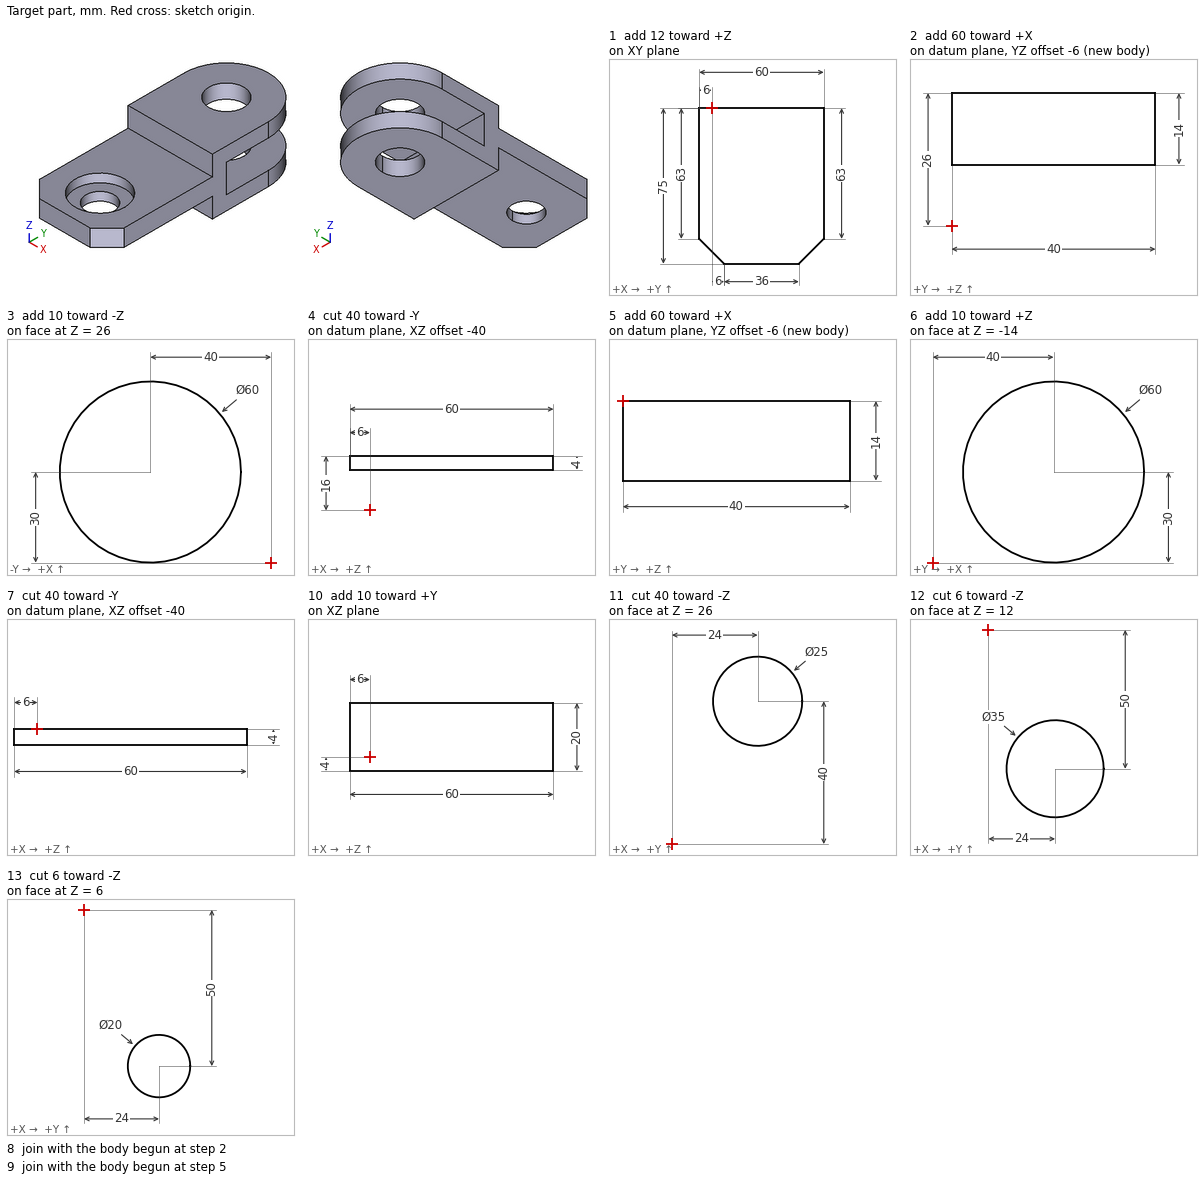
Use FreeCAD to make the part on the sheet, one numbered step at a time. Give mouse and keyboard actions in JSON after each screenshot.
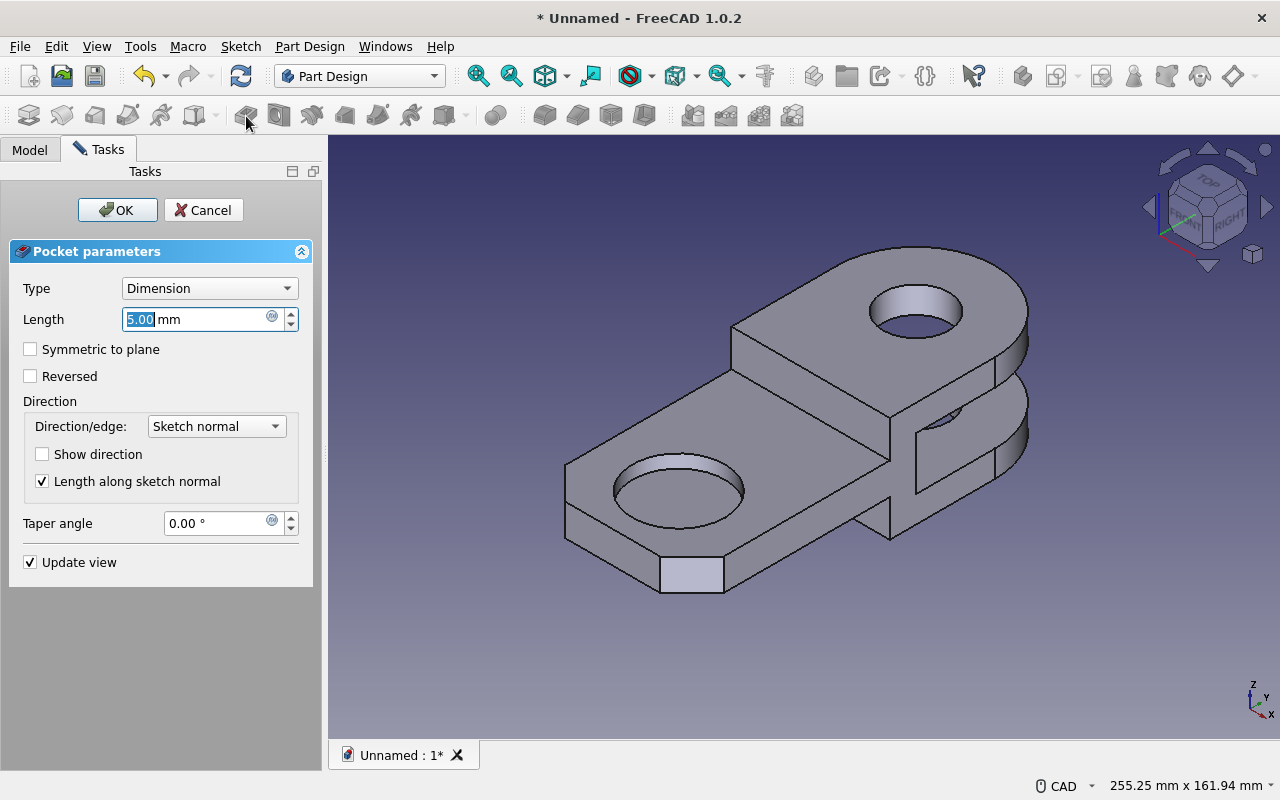
{"action": "type", "text": "6"}
{"action": "key", "text": "Tab"}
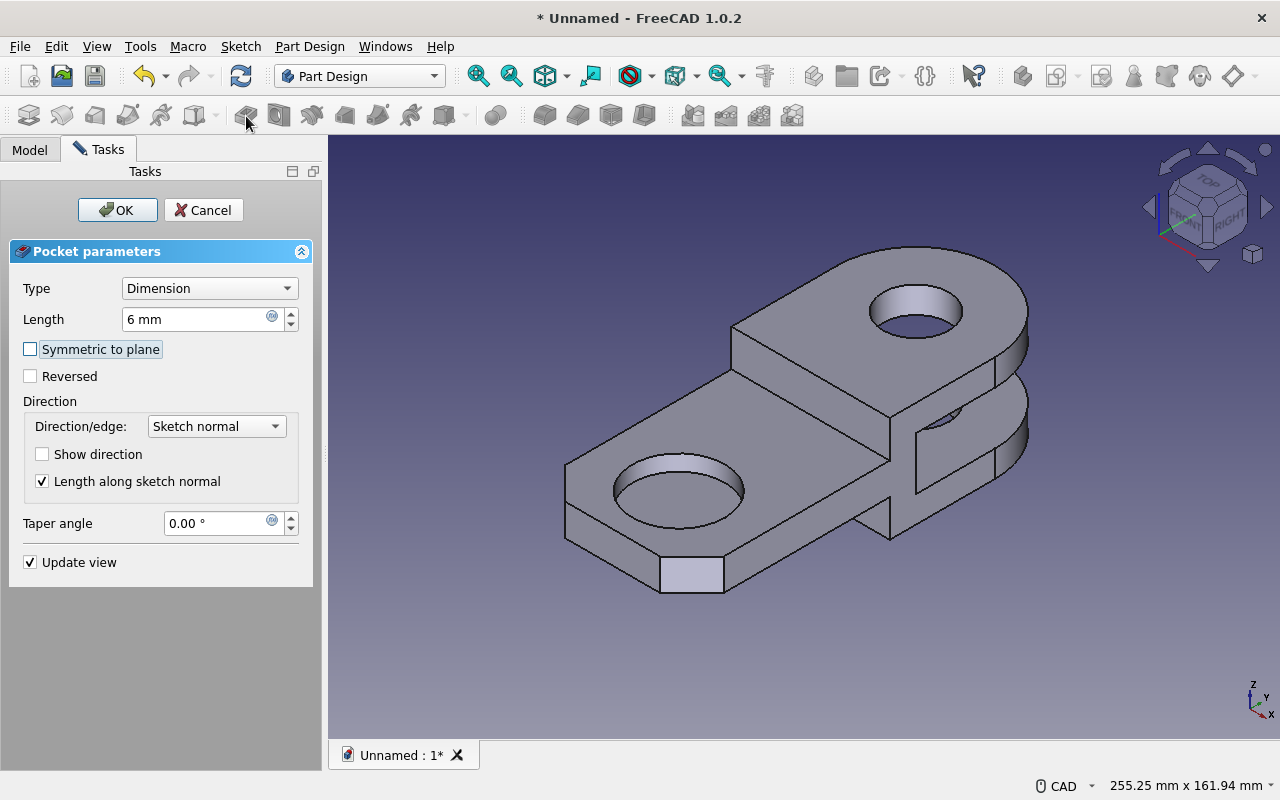
{"action": "left_click", "coordinate": [118, 210]}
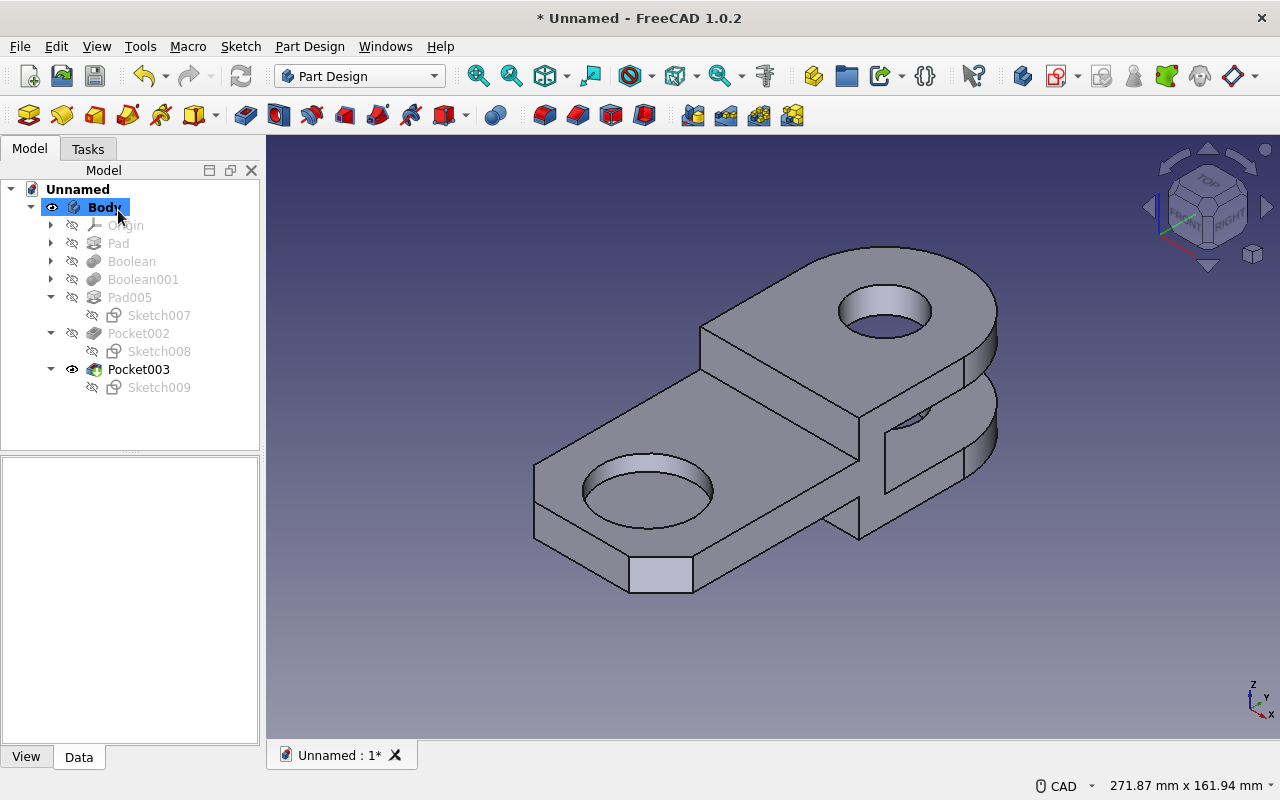
{"action": "left_click", "coordinate": [648, 508]}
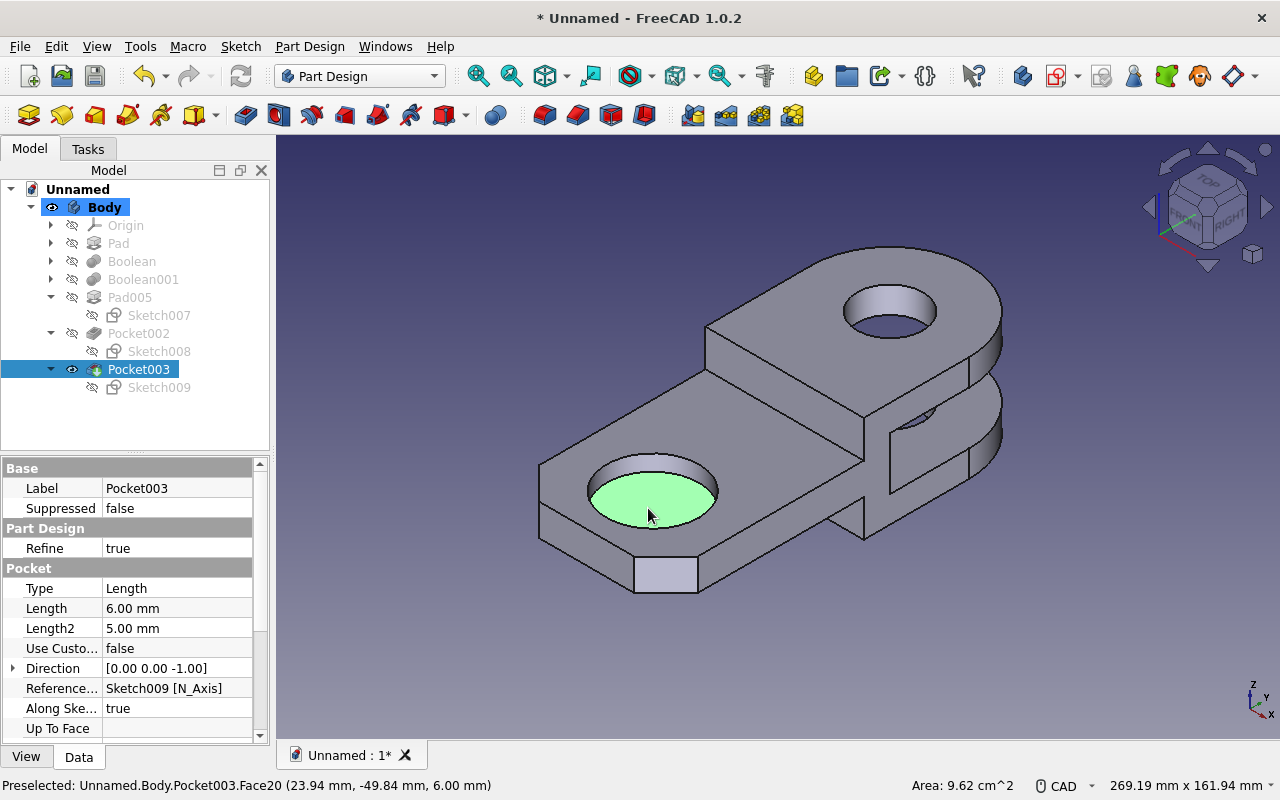
{"action": "left_click", "coordinate": [1056, 76]}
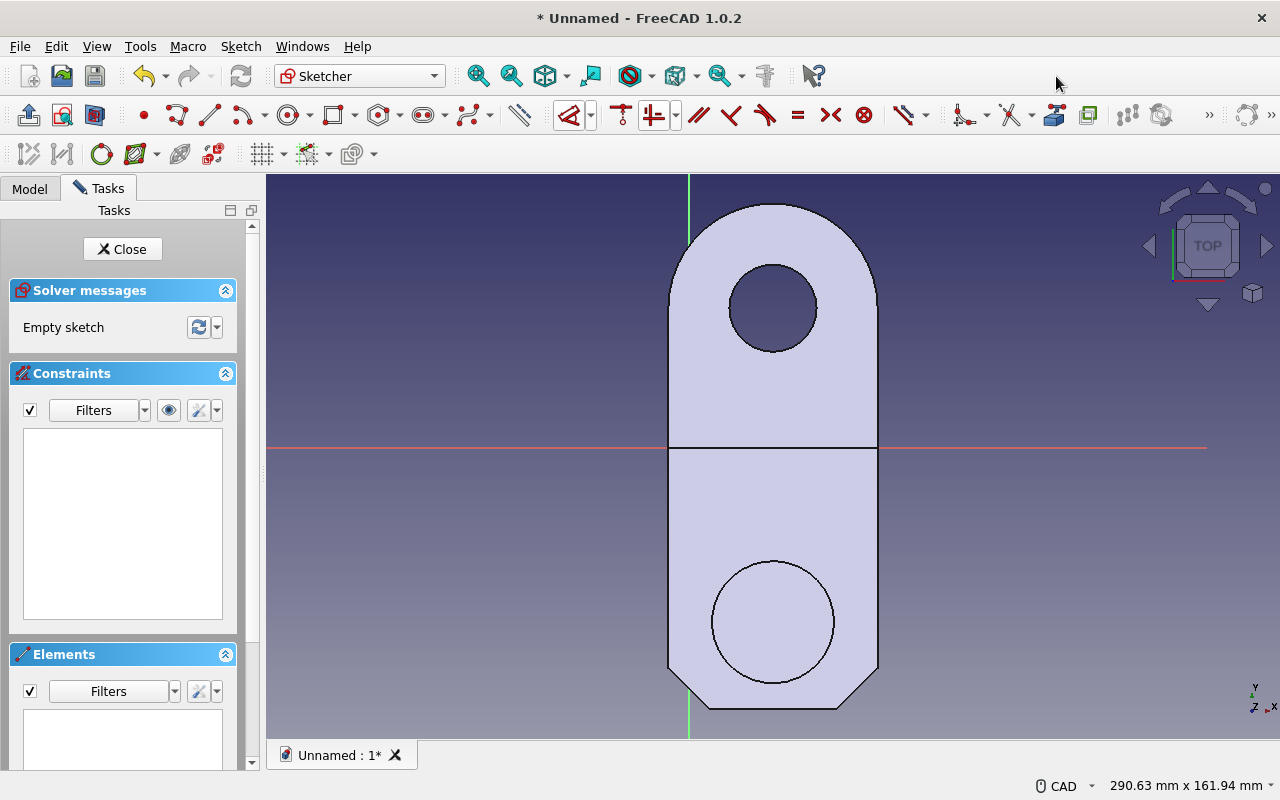
{"action": "left_click", "coordinate": [95, 116]}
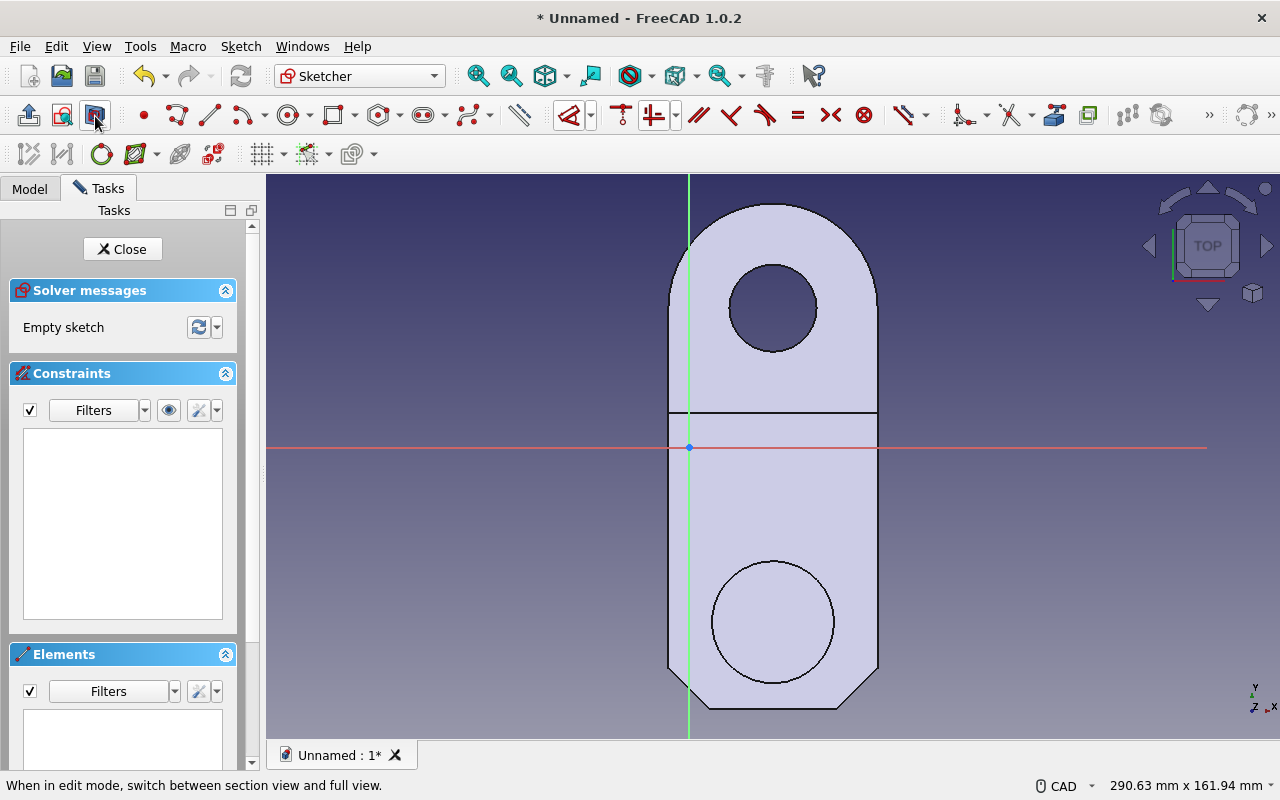
{"action": "scroll", "coordinate": [790, 664], "scroll_direction": "up", "scroll_amount": 8}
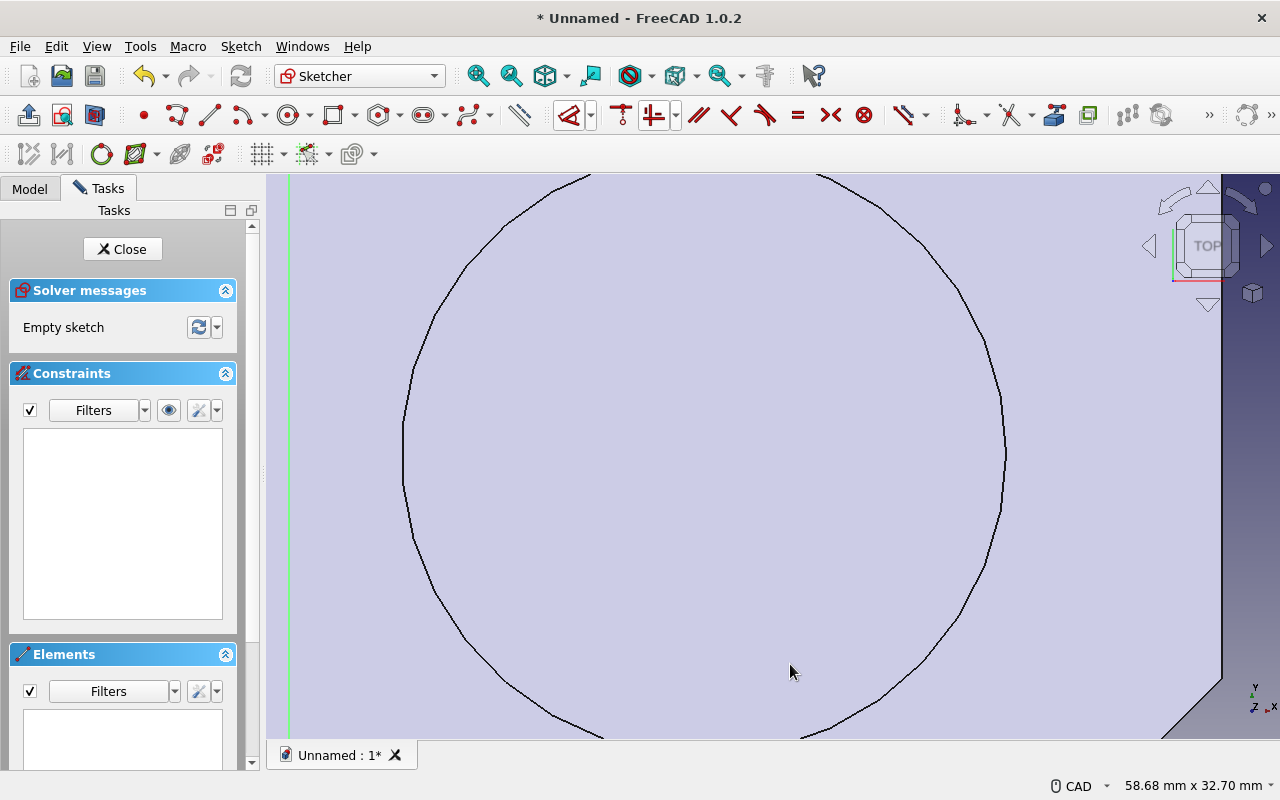
{"action": "left_click", "coordinate": [288, 116]}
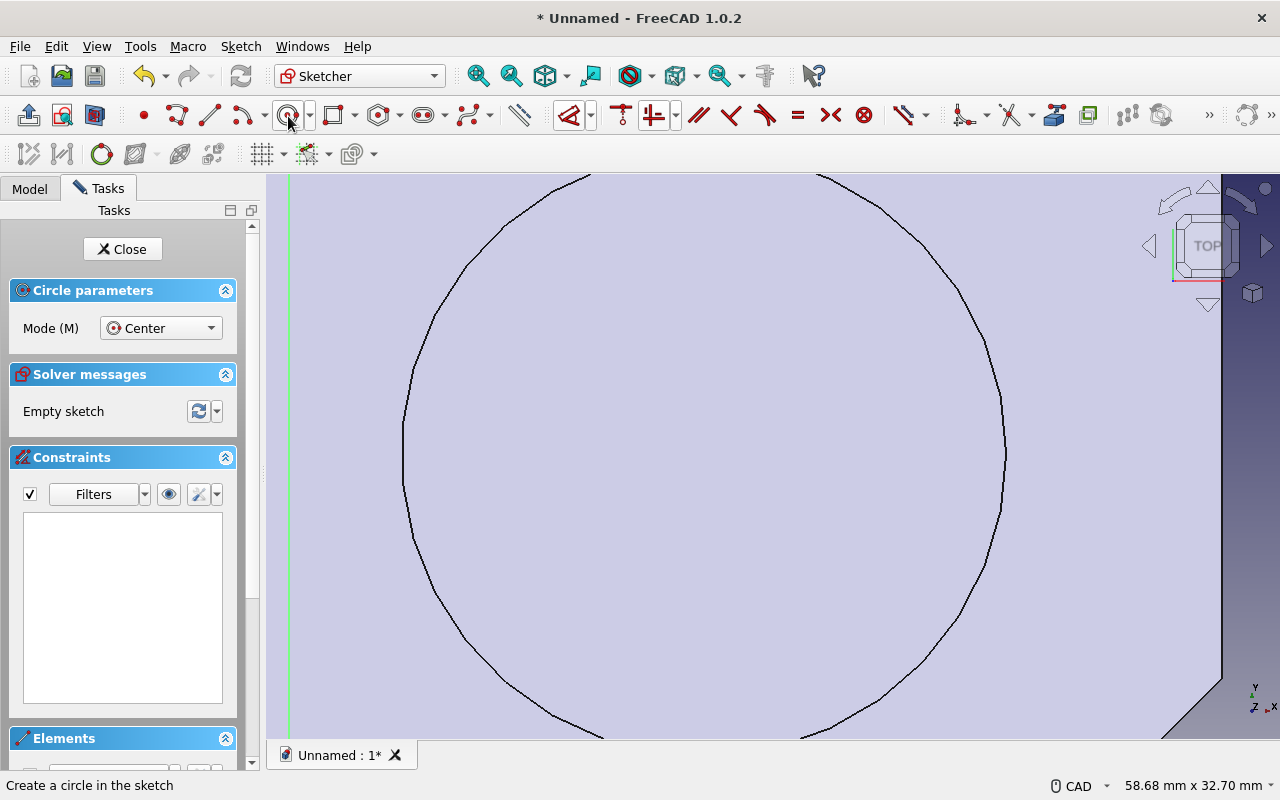
{"action": "left_click", "coordinate": [704, 454]}
{"action": "mouse_move", "coordinate": [826, 331]}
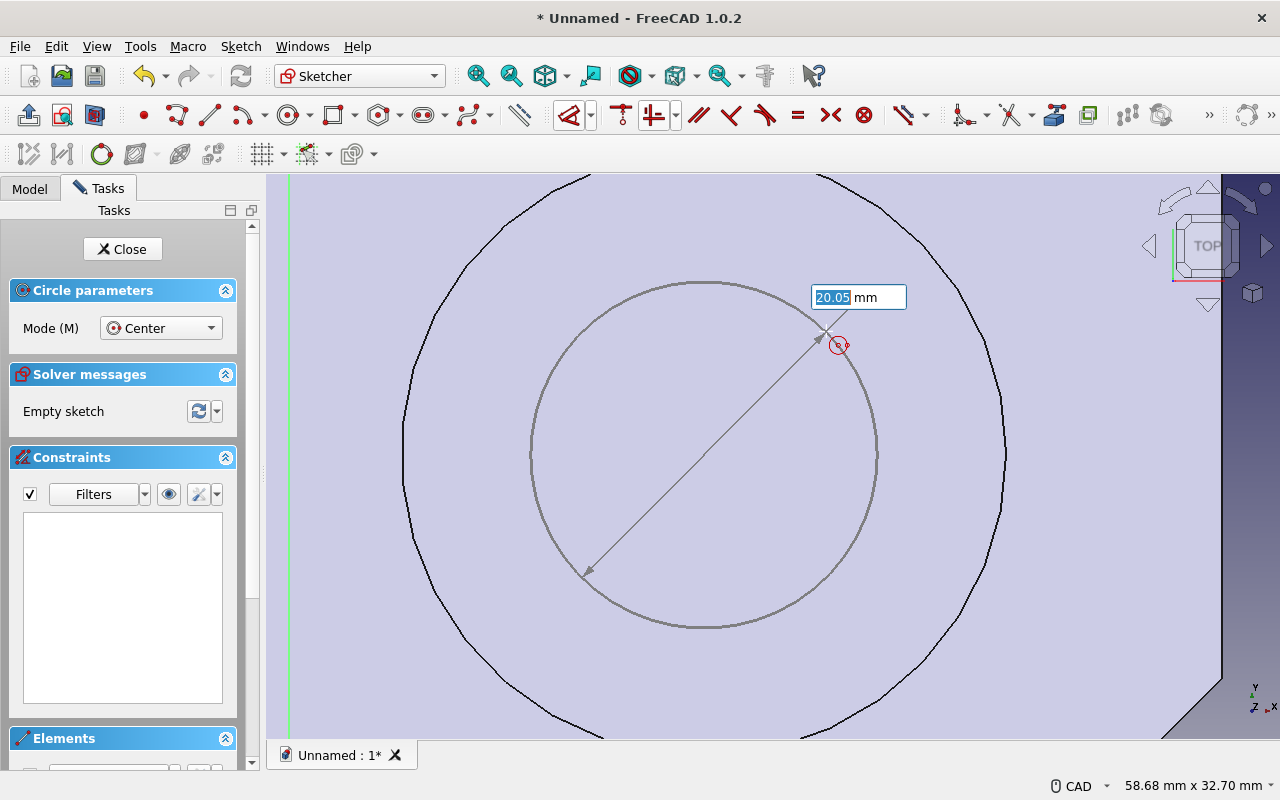
{"action": "type", "text": "20"}
{"action": "key", "text": "Return"}
{"action": "key", "text": "Escape"}